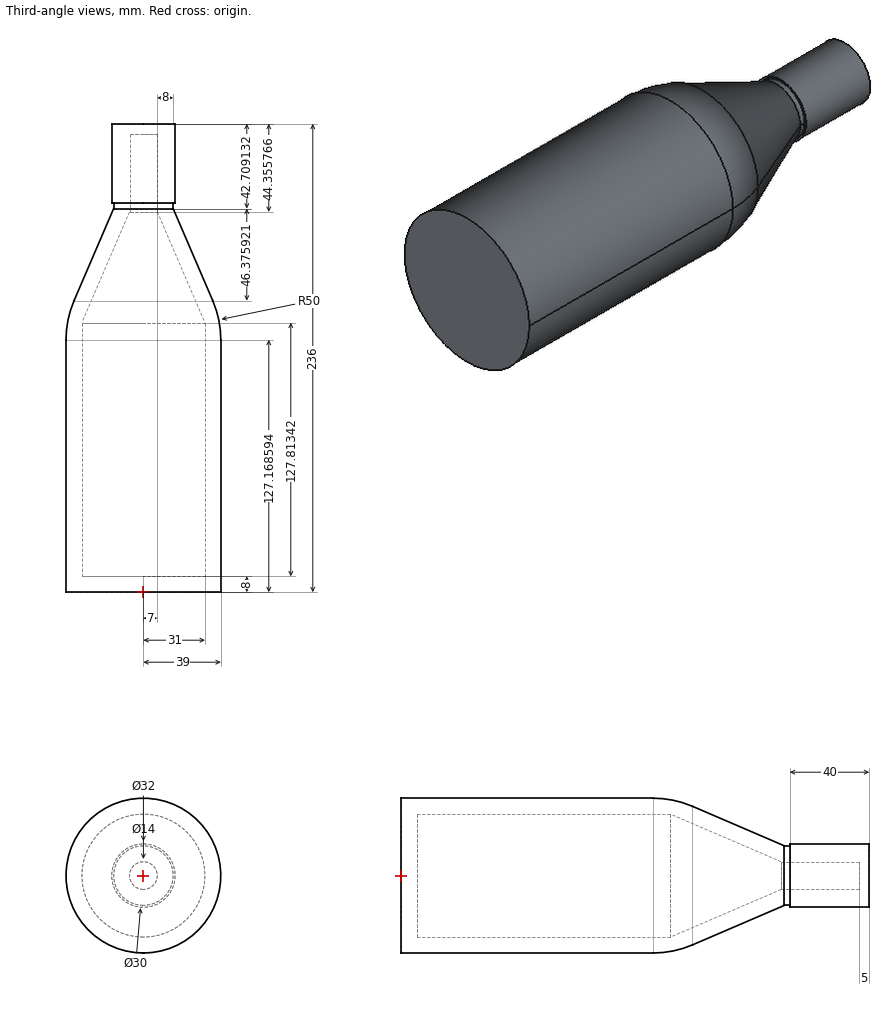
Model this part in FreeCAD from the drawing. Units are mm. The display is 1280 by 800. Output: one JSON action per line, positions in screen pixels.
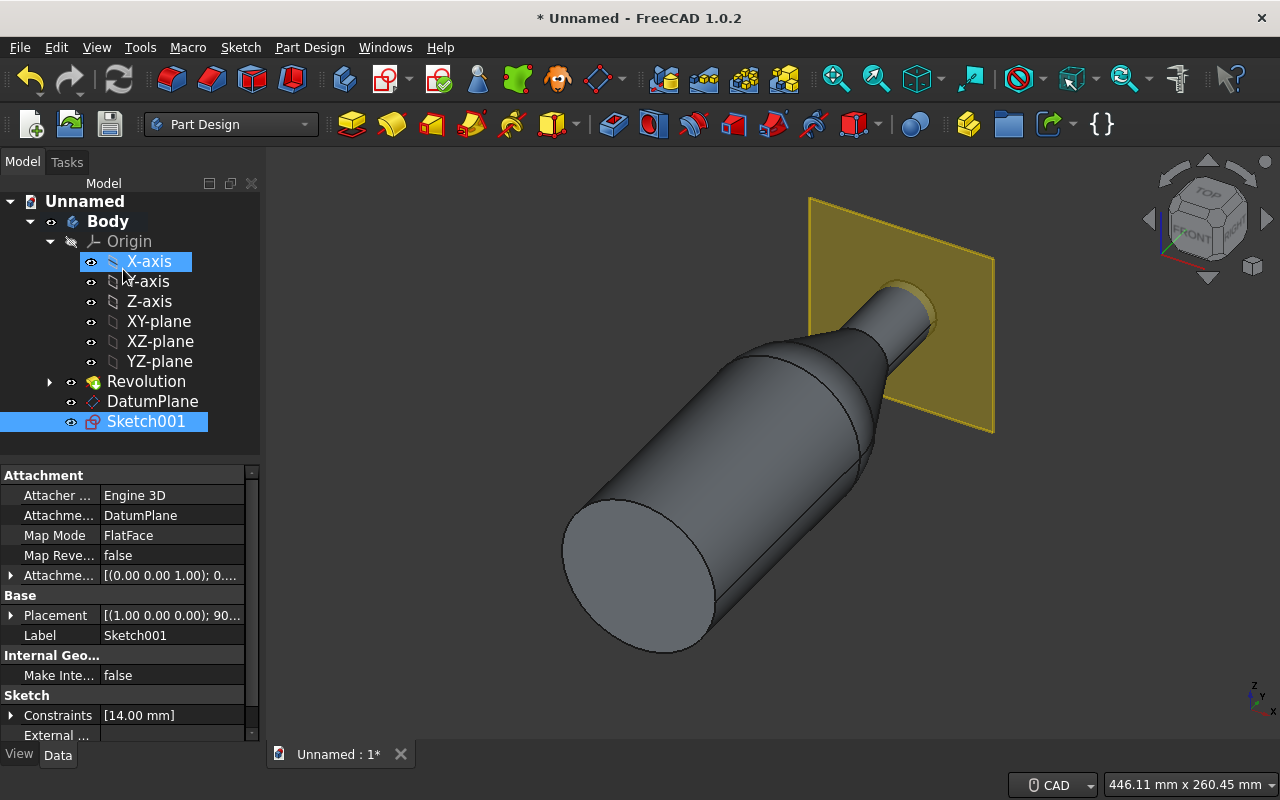
{"action": "left_click", "coordinate": [352, 124]}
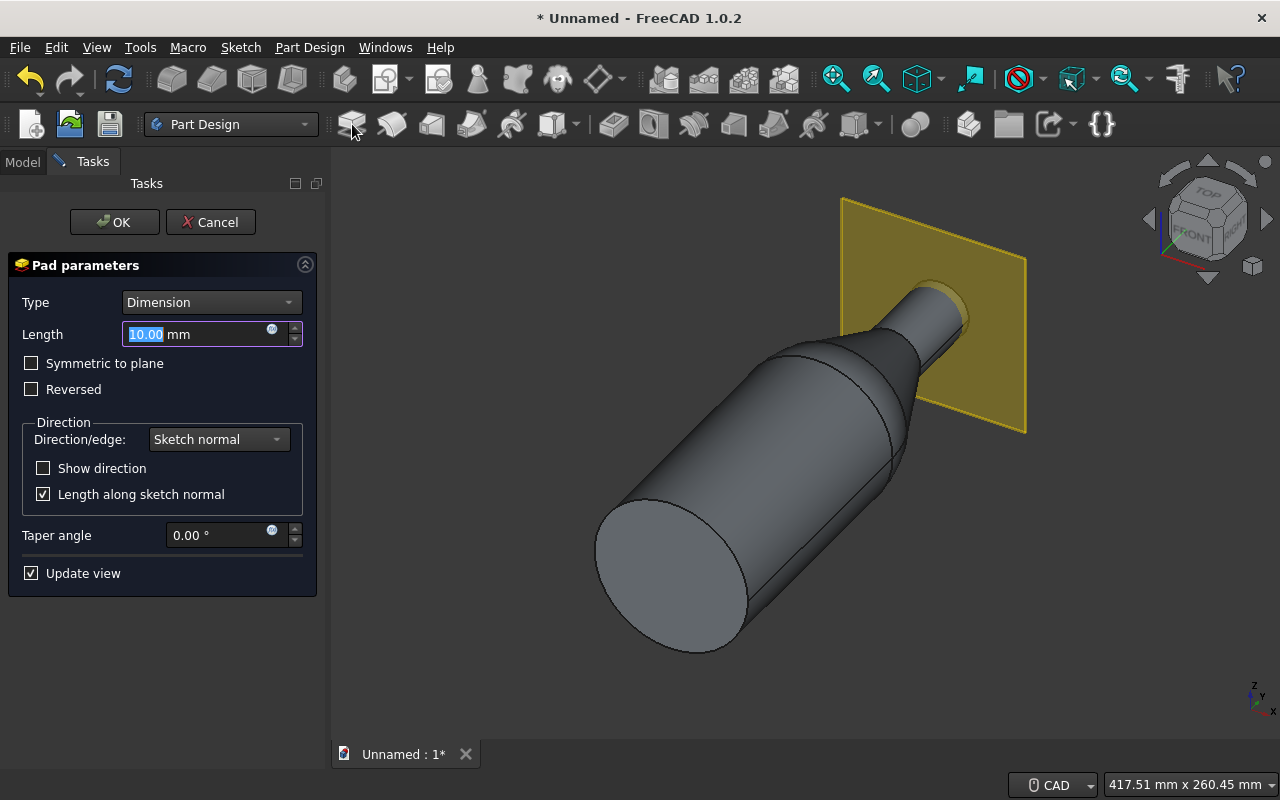
{"action": "type", "text": "5"}
{"action": "key", "text": "Tab"}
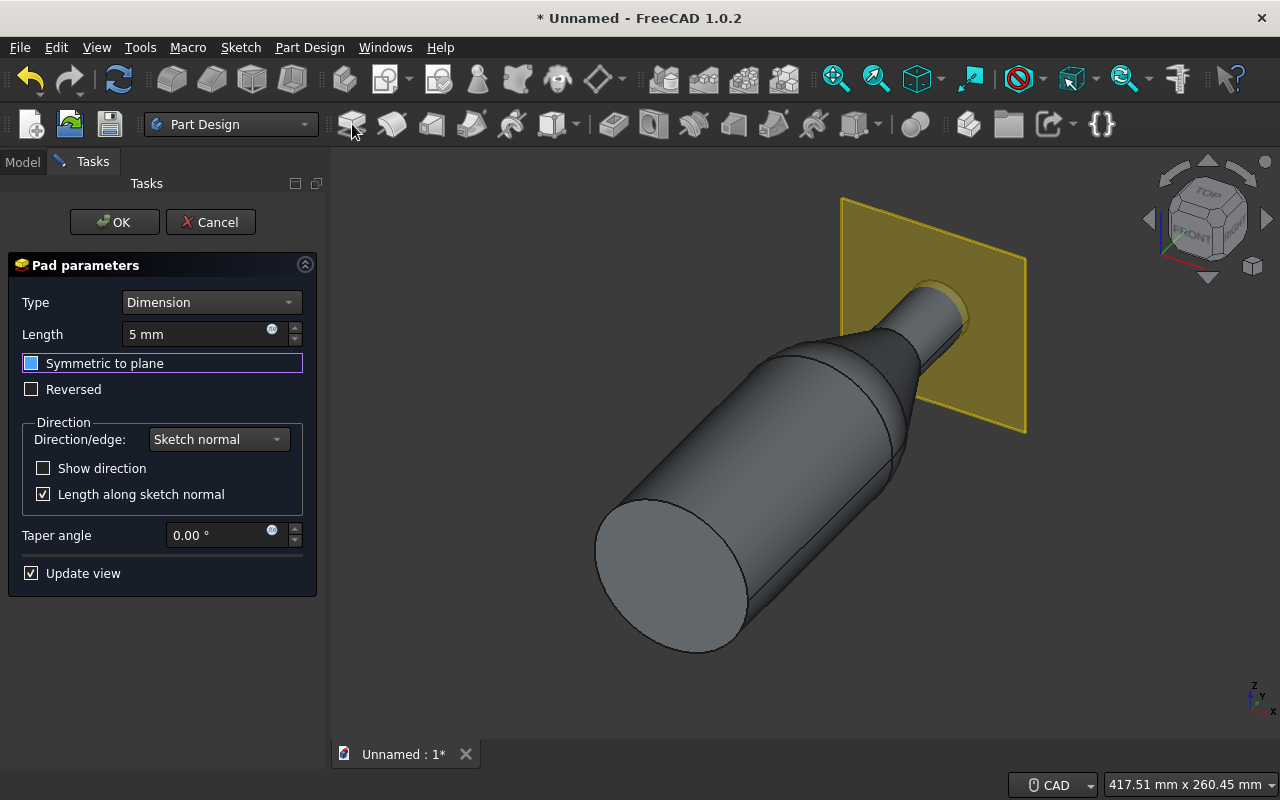
{"action": "left_click", "coordinate": [30, 389]}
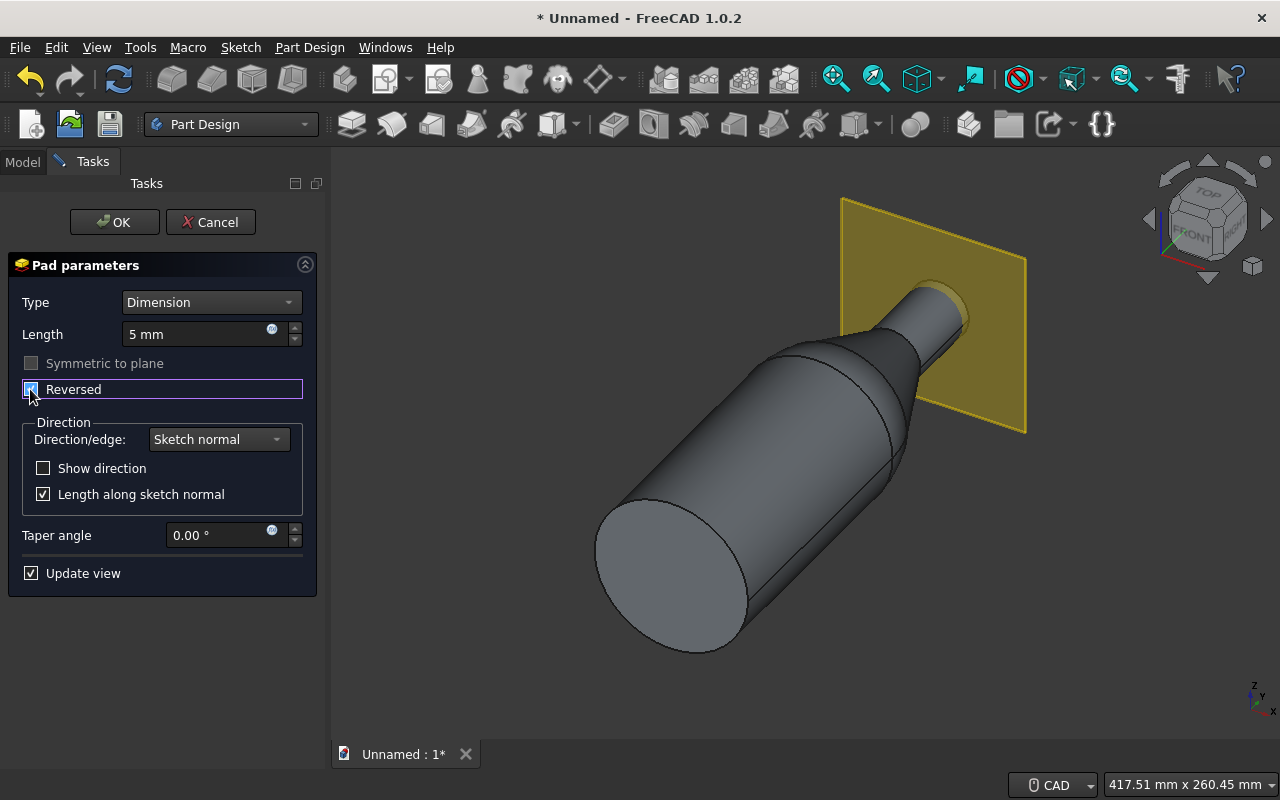
{"action": "left_click", "coordinate": [115, 222]}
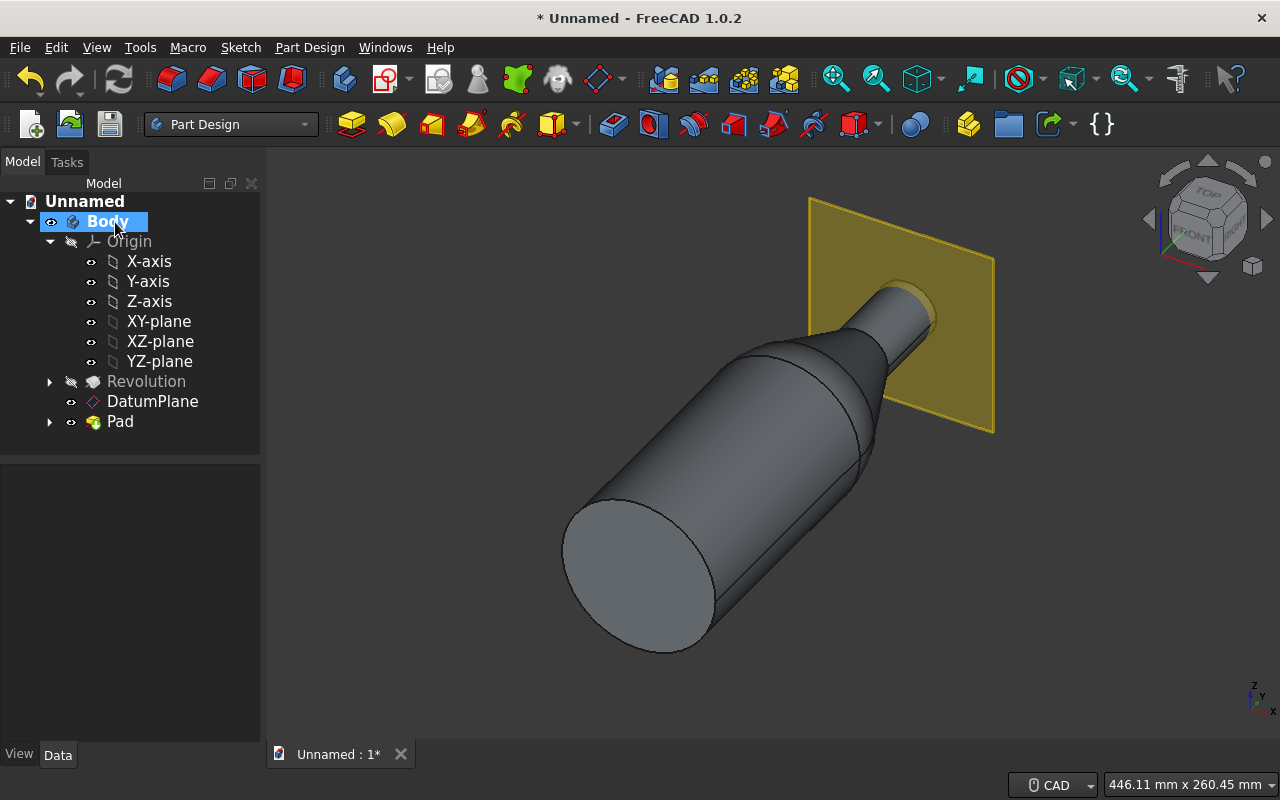
{"action": "left_click", "coordinate": [116, 402]}
{"action": "key", "text": "space"}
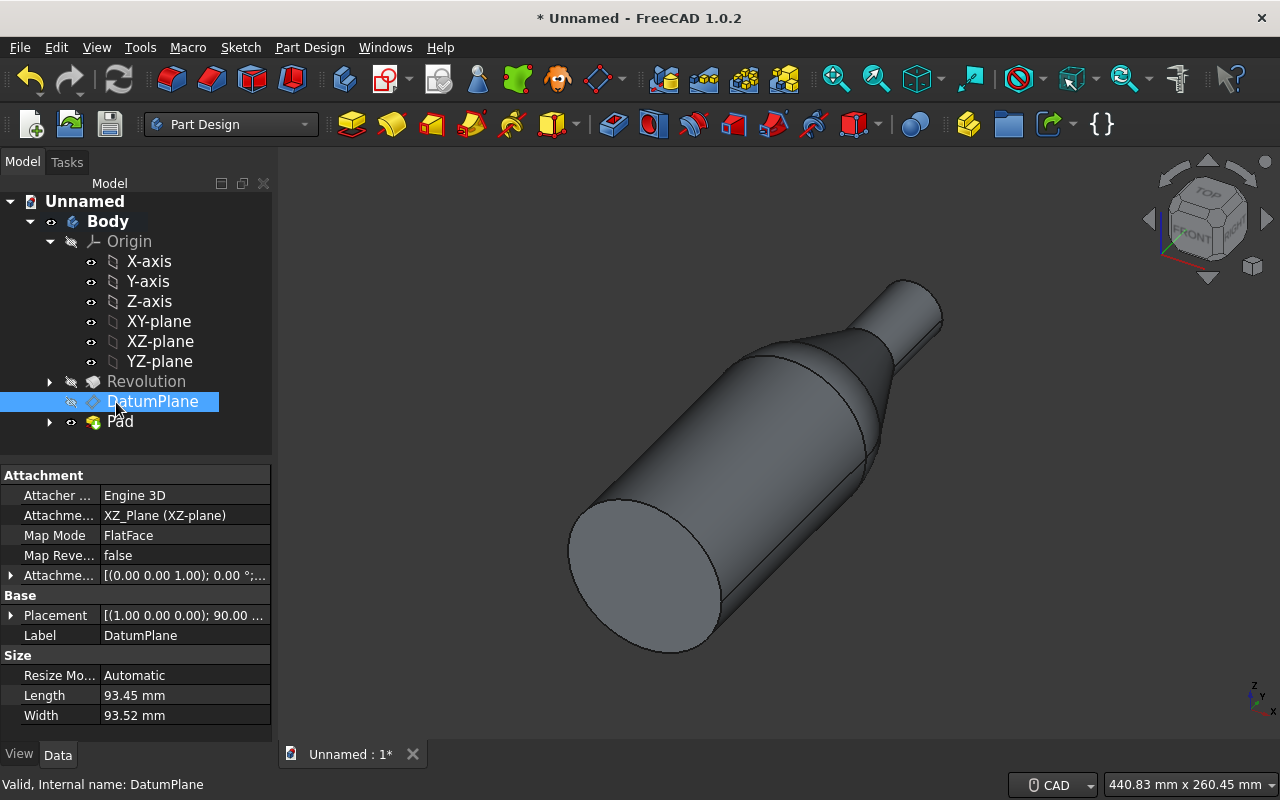
{"action": "key", "text": "4"}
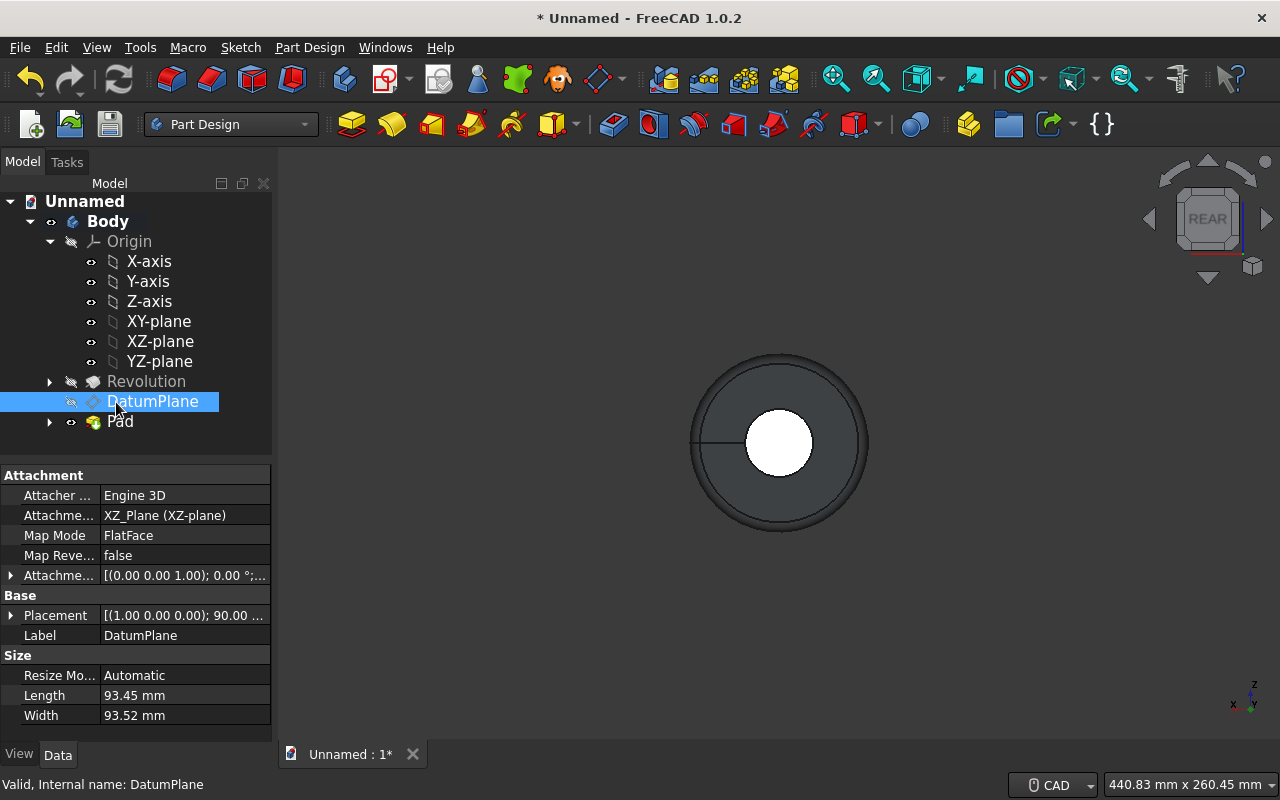
{"action": "key", "text": "v f"}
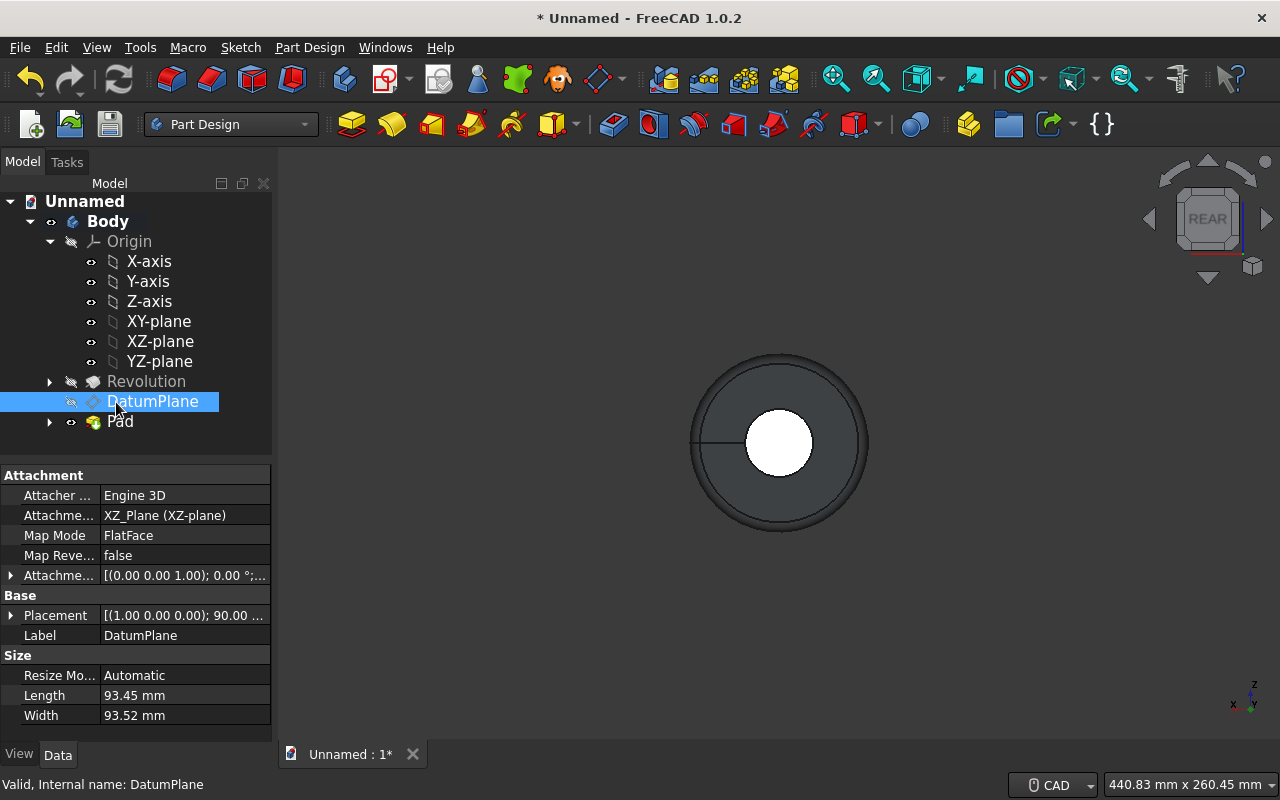
{"action": "left_click", "coordinate": [779, 442]}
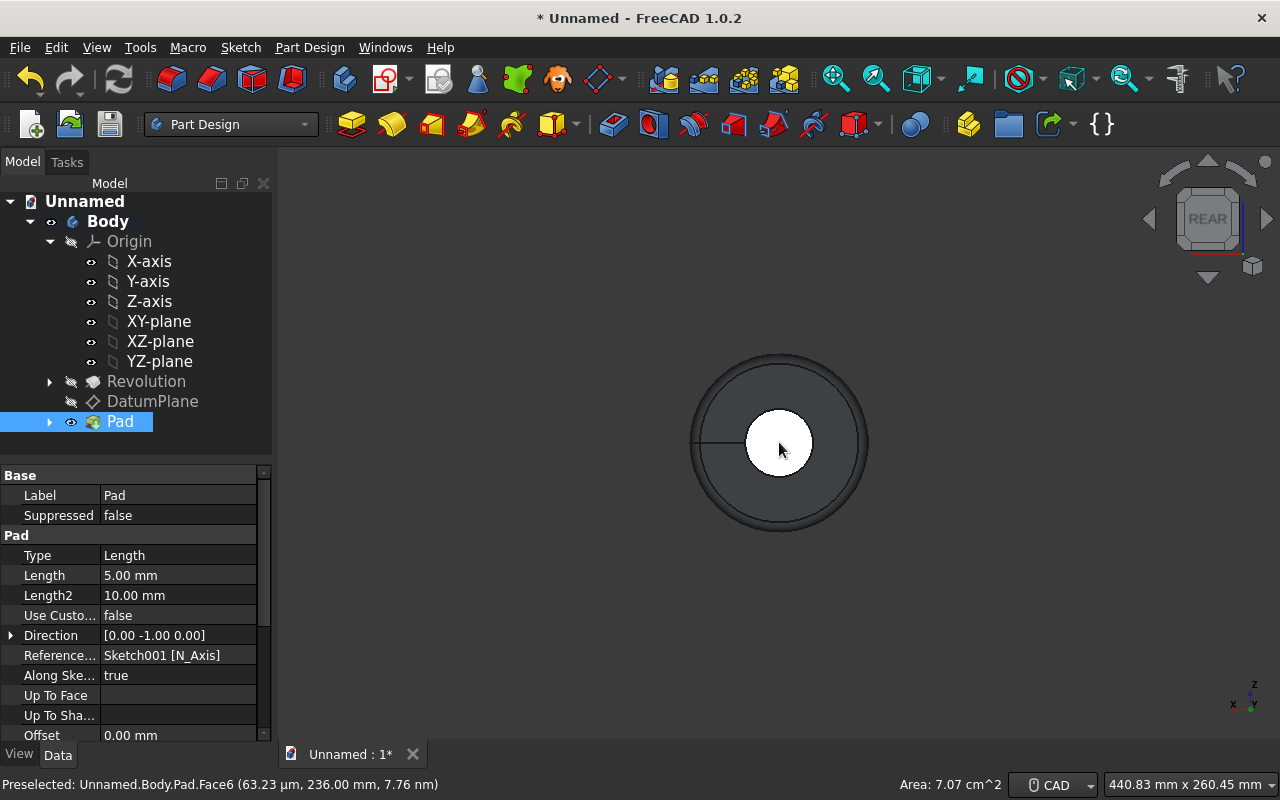
{"action": "left_click", "coordinate": [386, 80]}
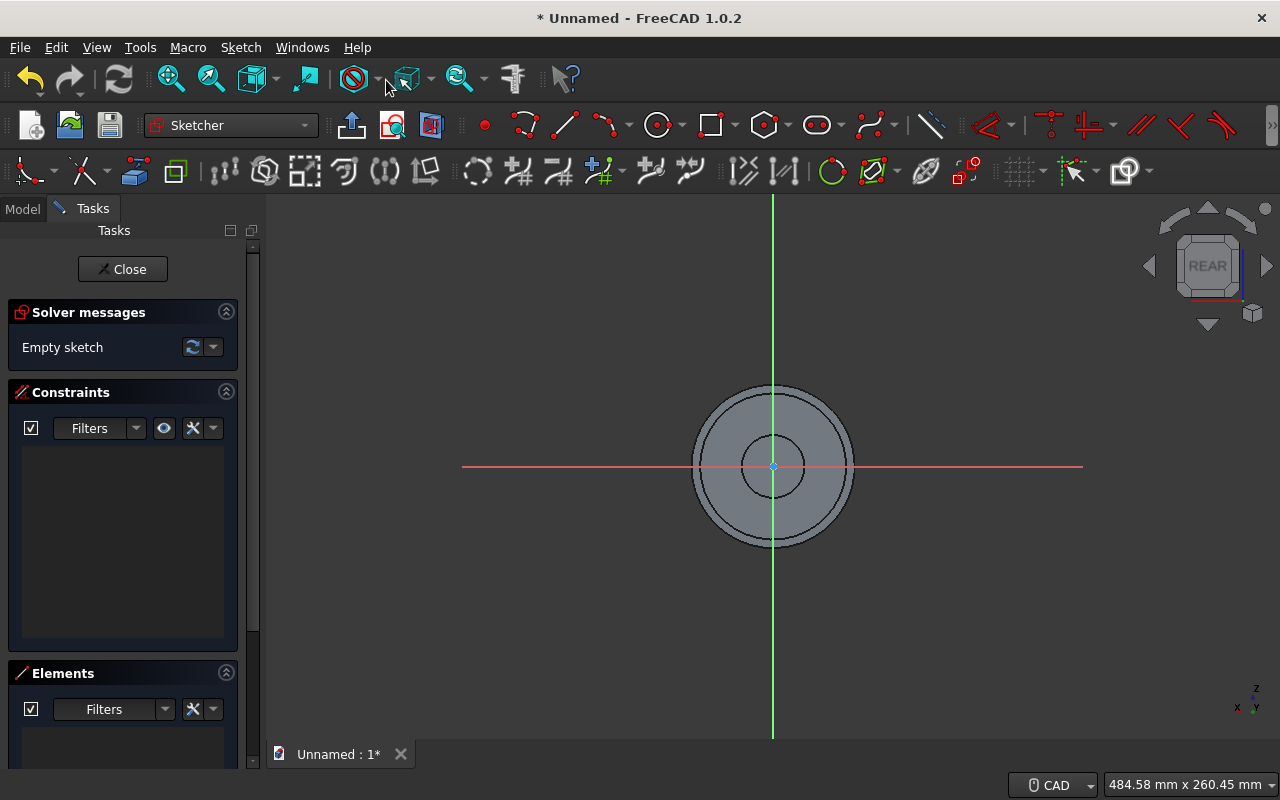
{"action": "scroll", "coordinate": [790, 466], "scroll_direction": "up", "scroll_amount": 8}